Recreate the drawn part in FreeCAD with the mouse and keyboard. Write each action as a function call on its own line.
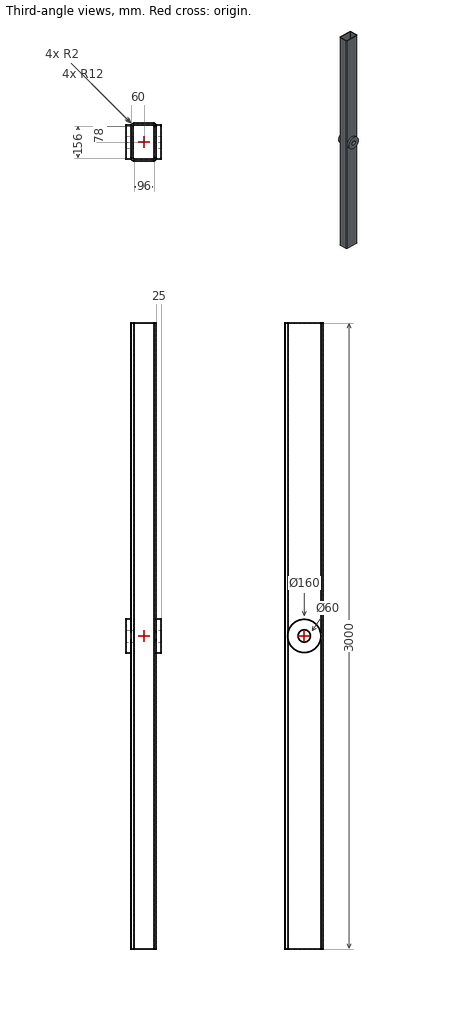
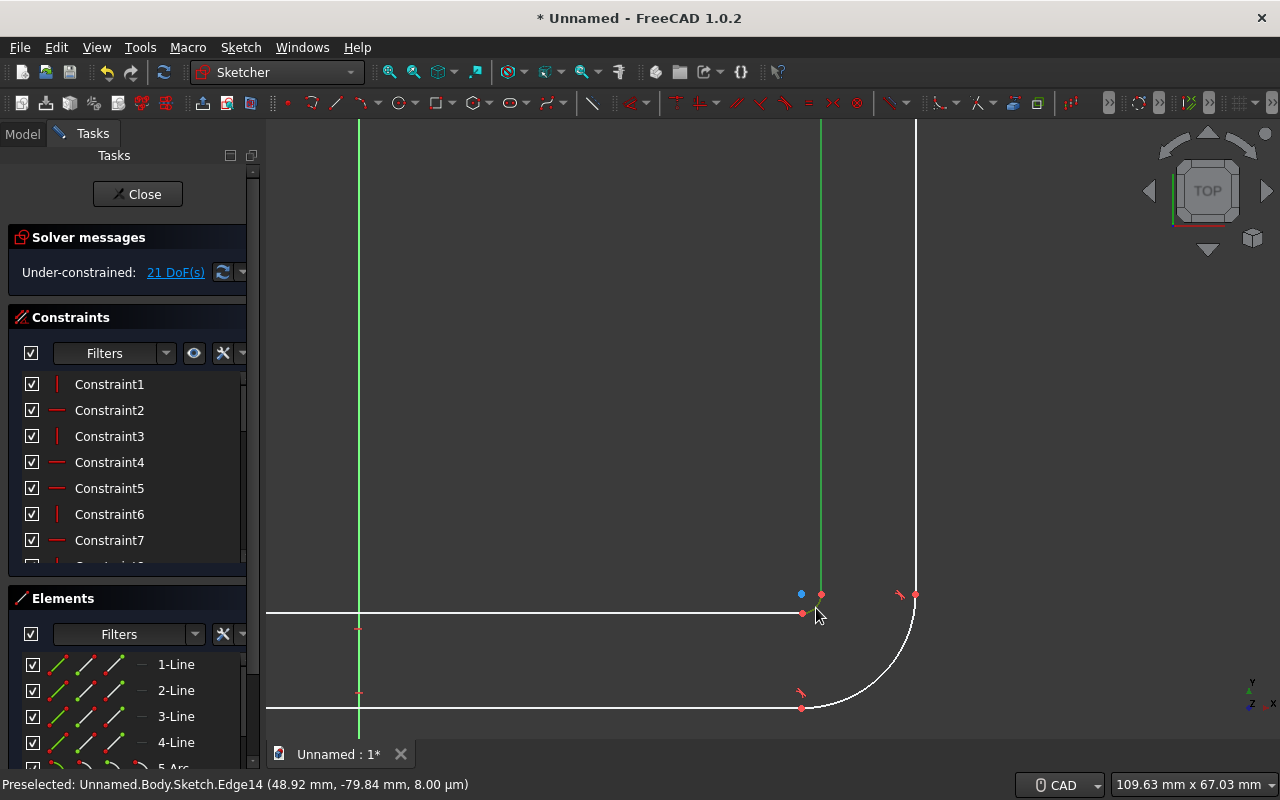
click(786, 104)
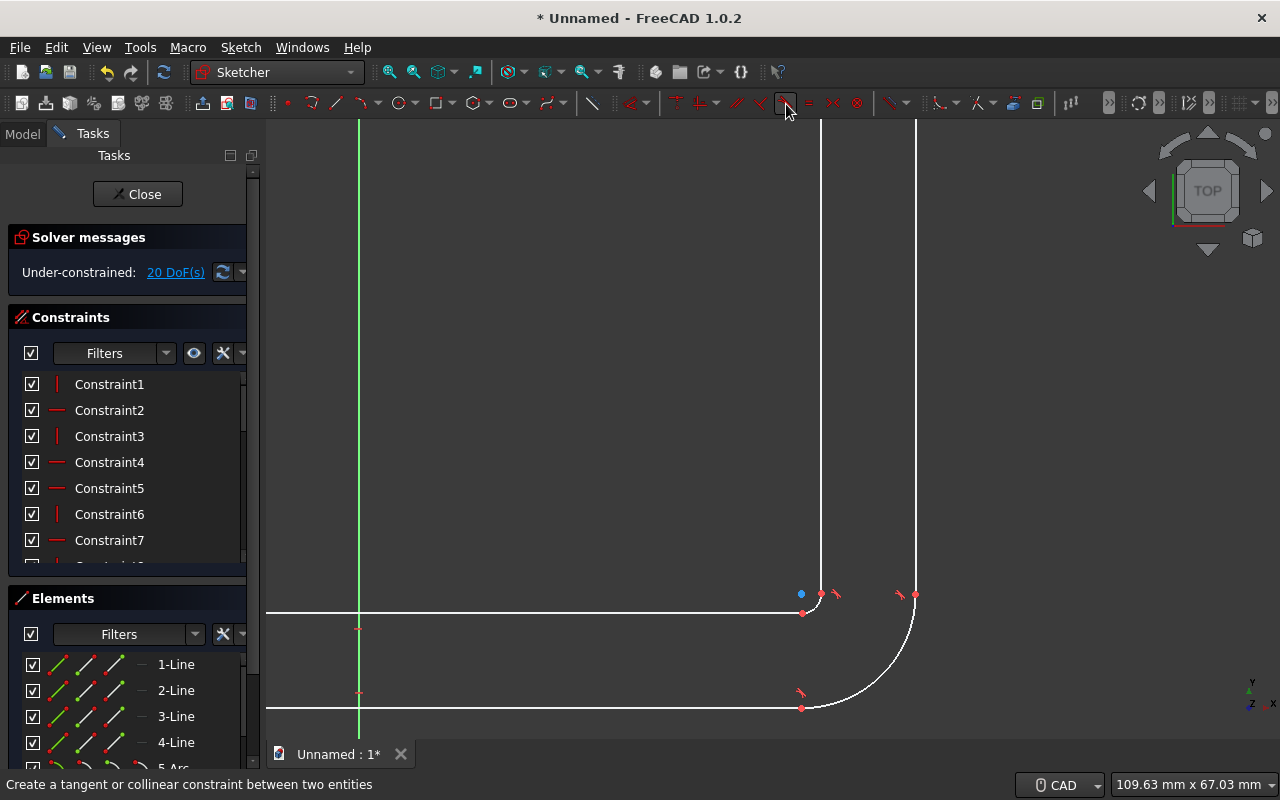
scroll(818, 611, down, 7)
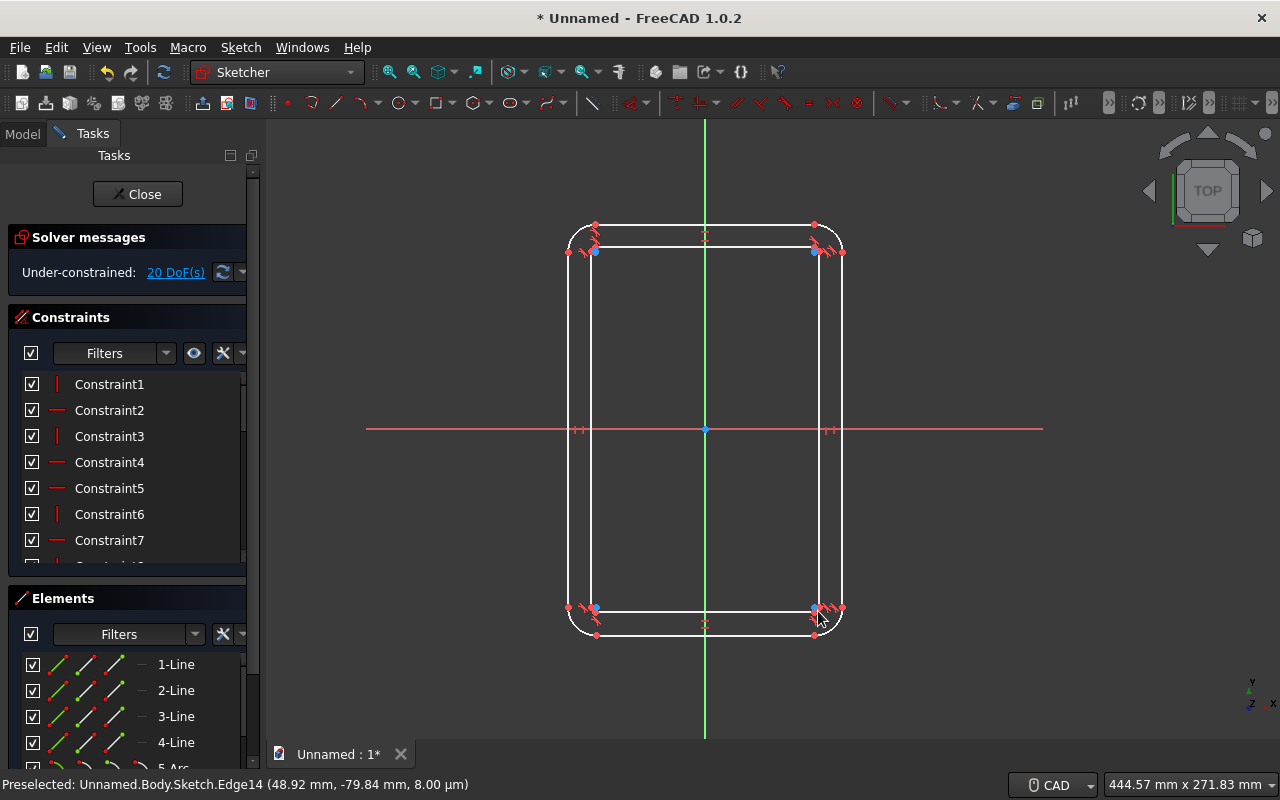
click(749, 612)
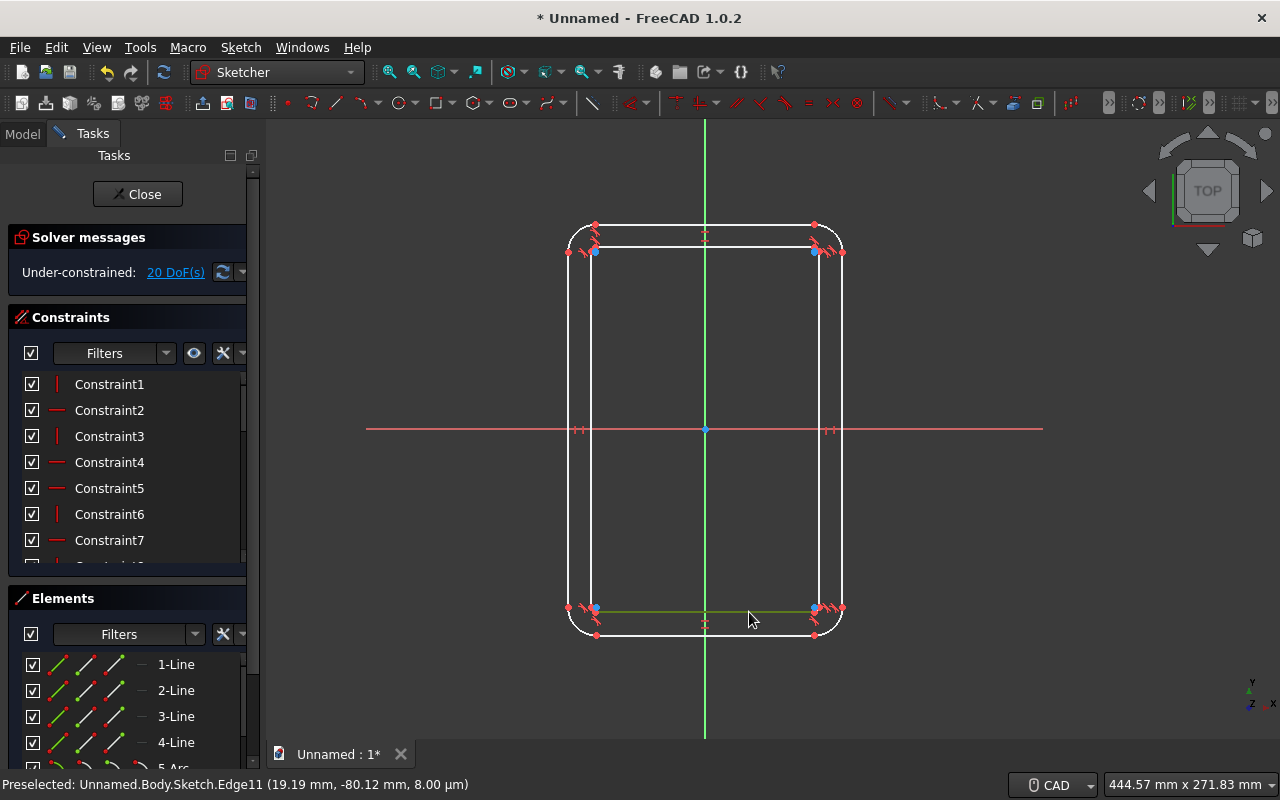
scroll(818, 611, up, 7)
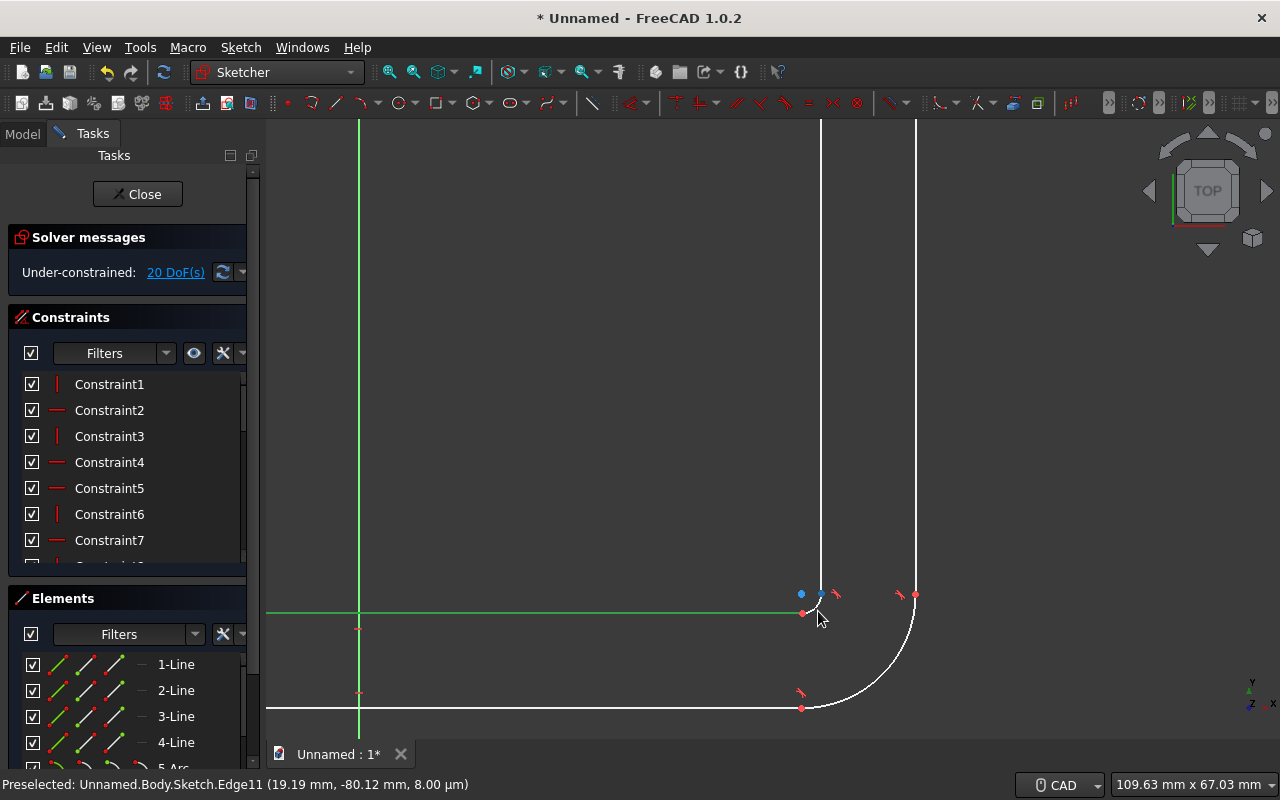
click(816, 607)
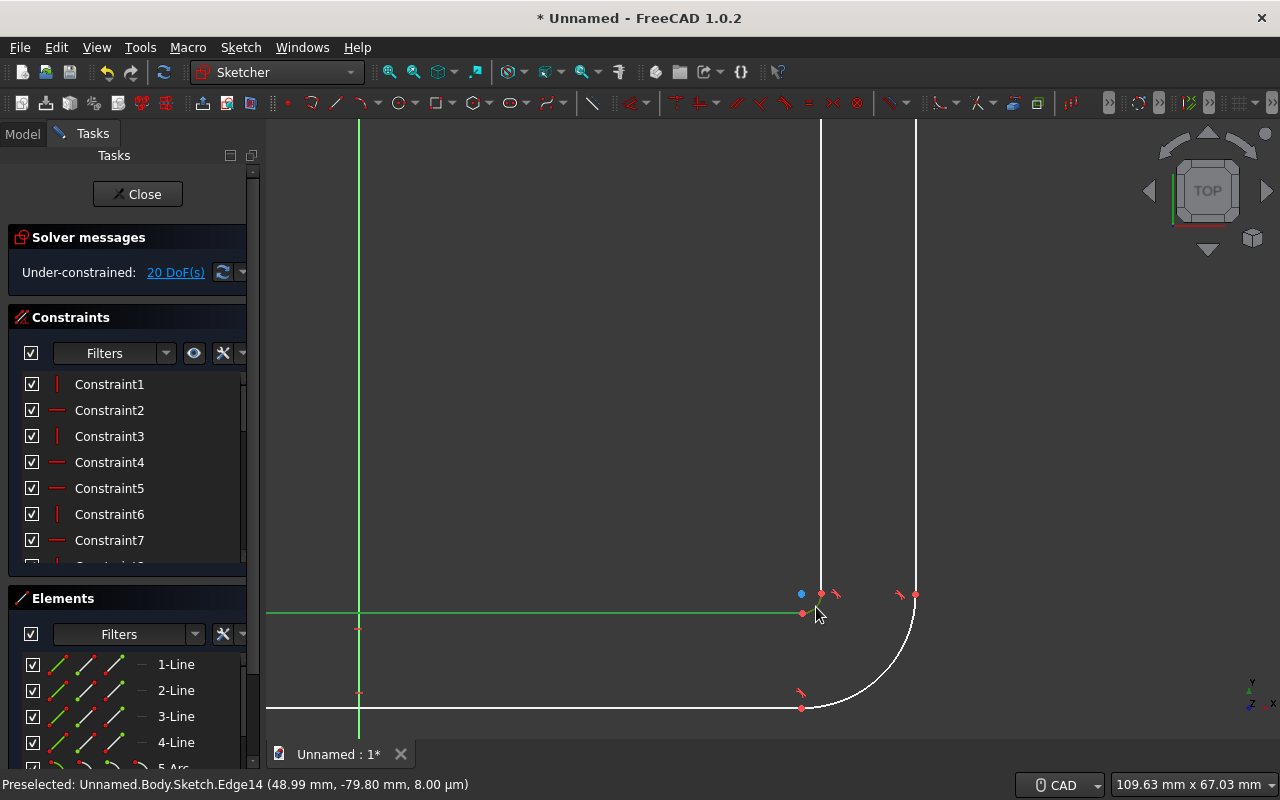
click(786, 104)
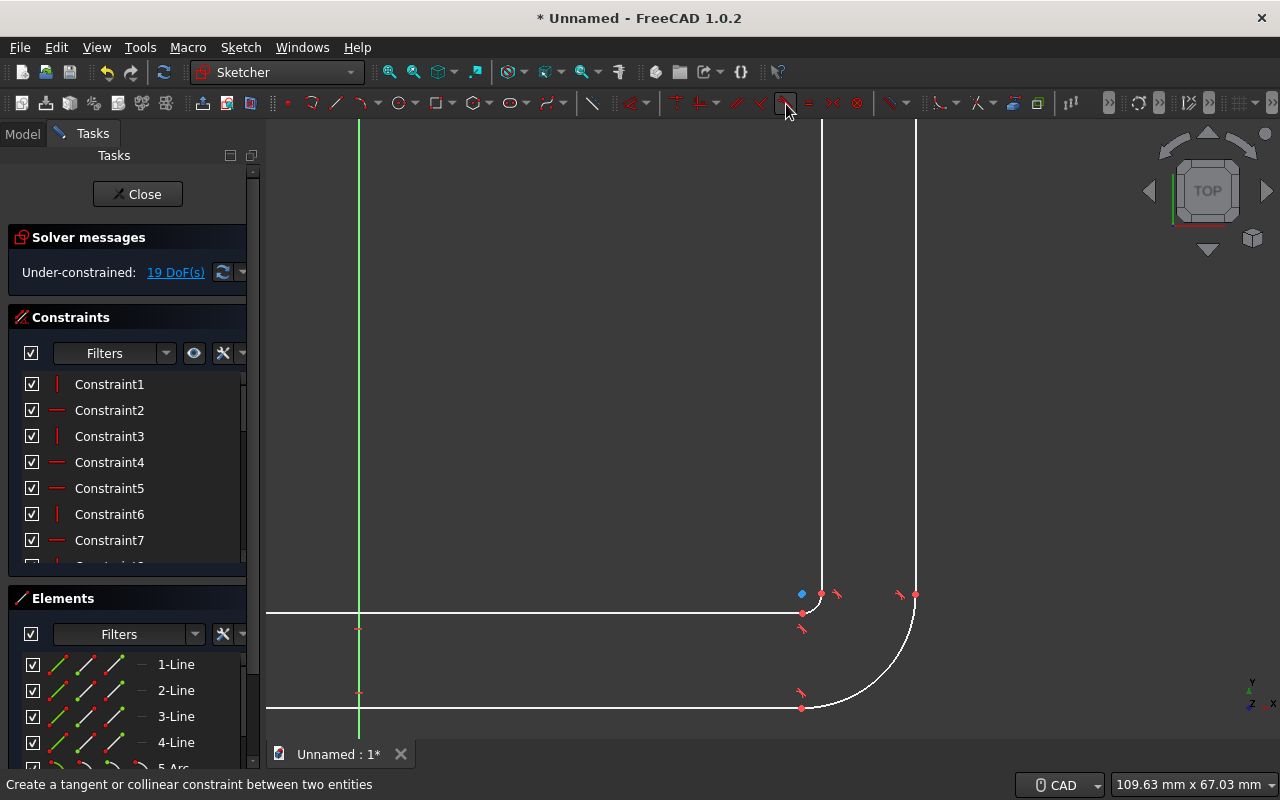
scroll(818, 611, down, 7)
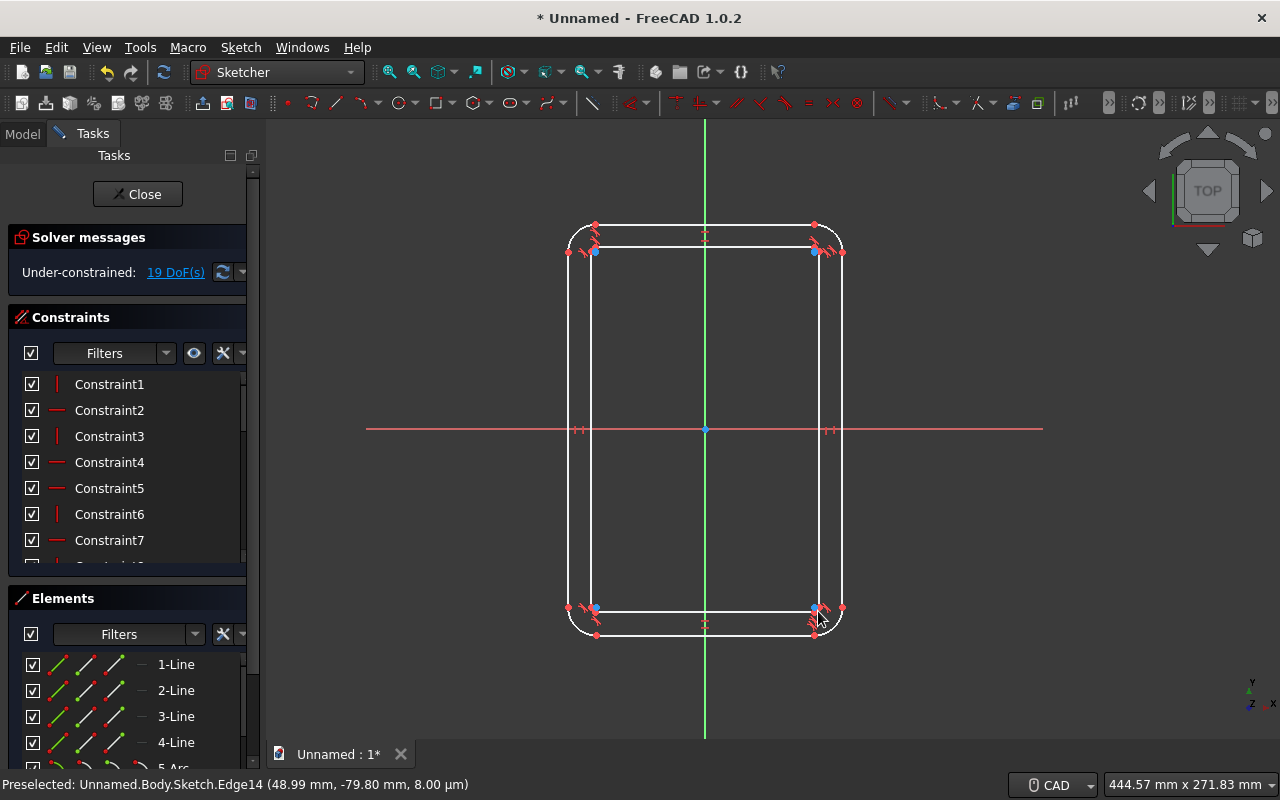
click(749, 612)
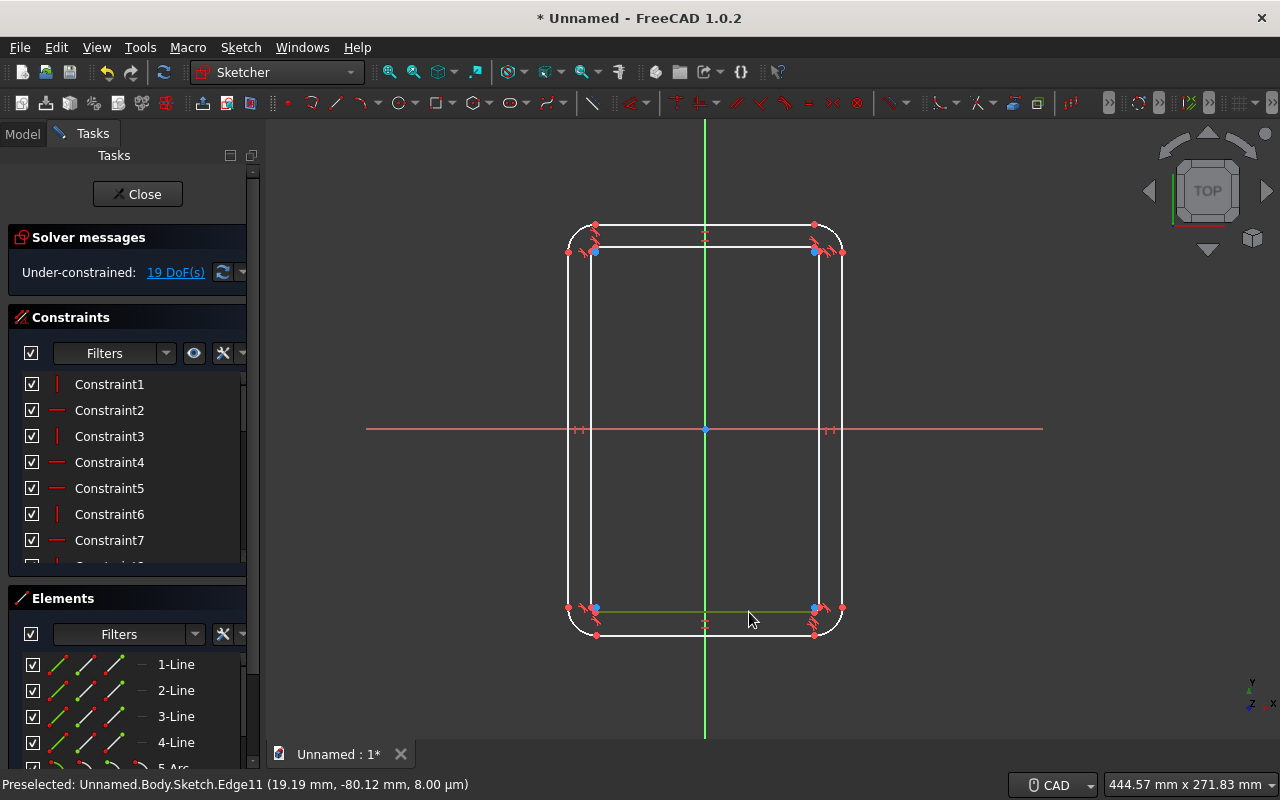
scroll(593, 611, up, 7)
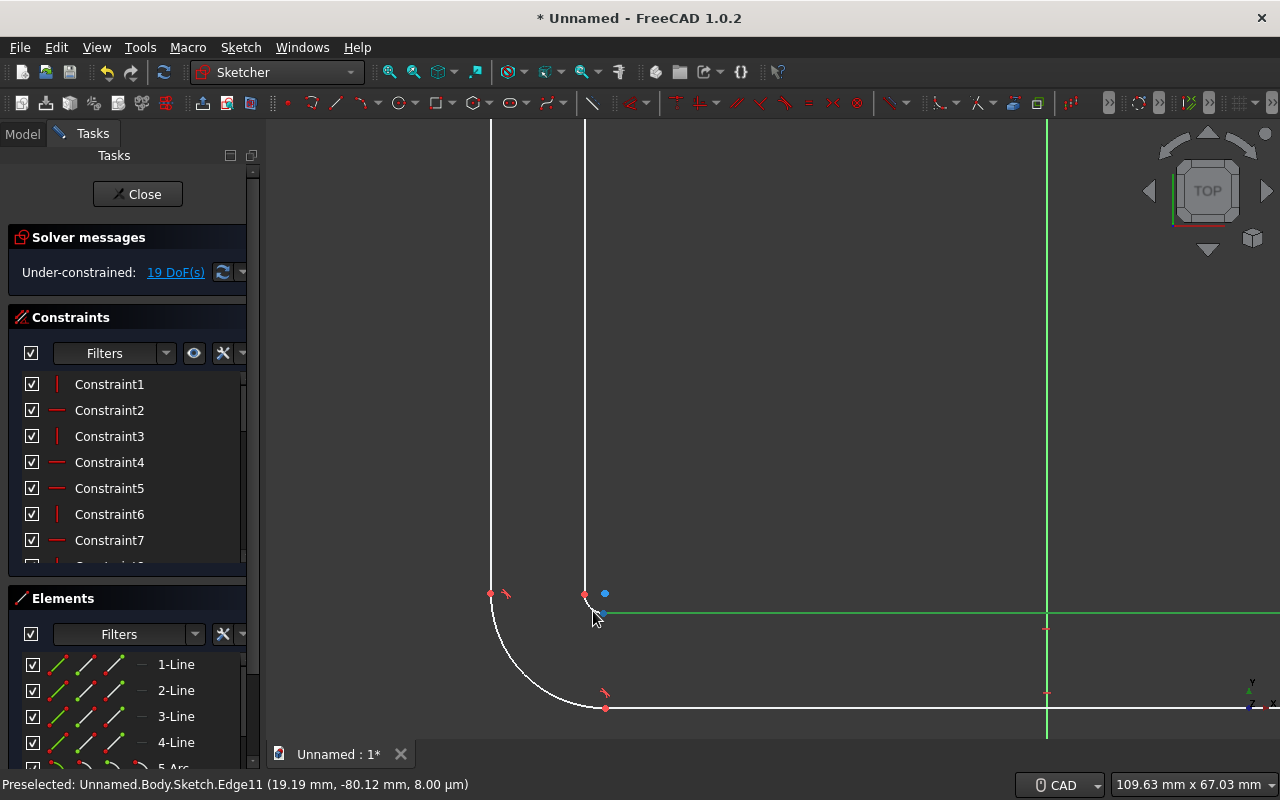
click(591, 608)